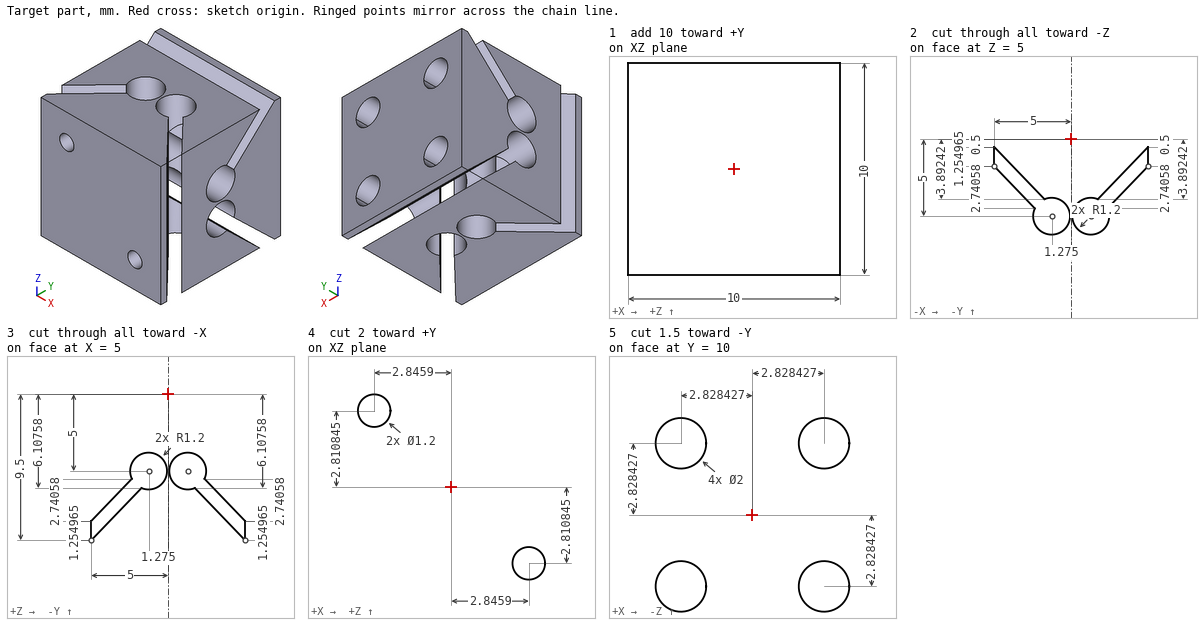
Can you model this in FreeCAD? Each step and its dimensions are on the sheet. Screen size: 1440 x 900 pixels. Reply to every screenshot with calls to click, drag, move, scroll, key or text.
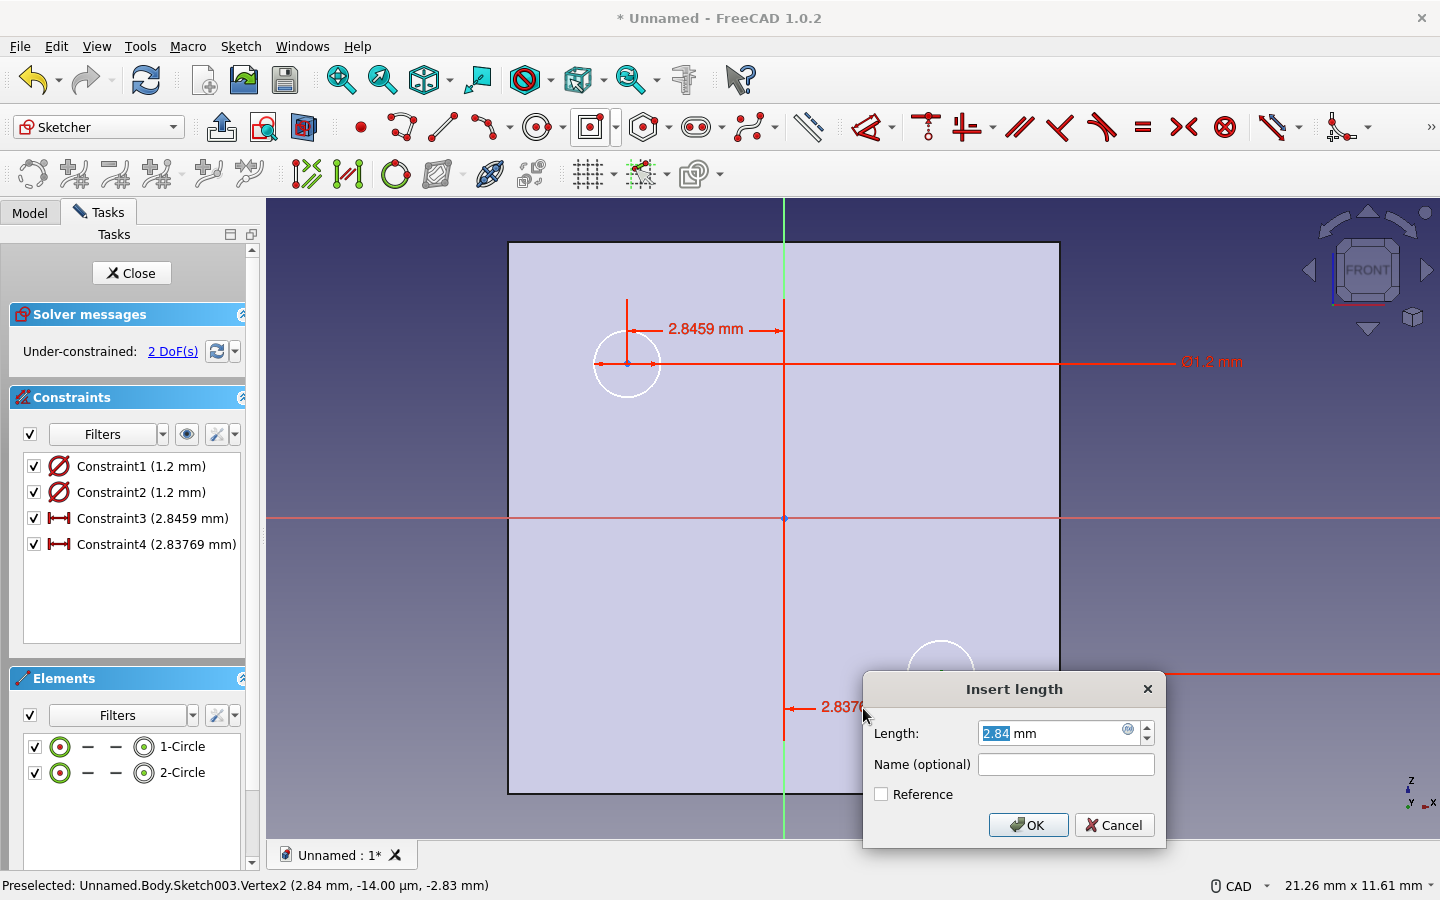
text(2.8459)
key(Return)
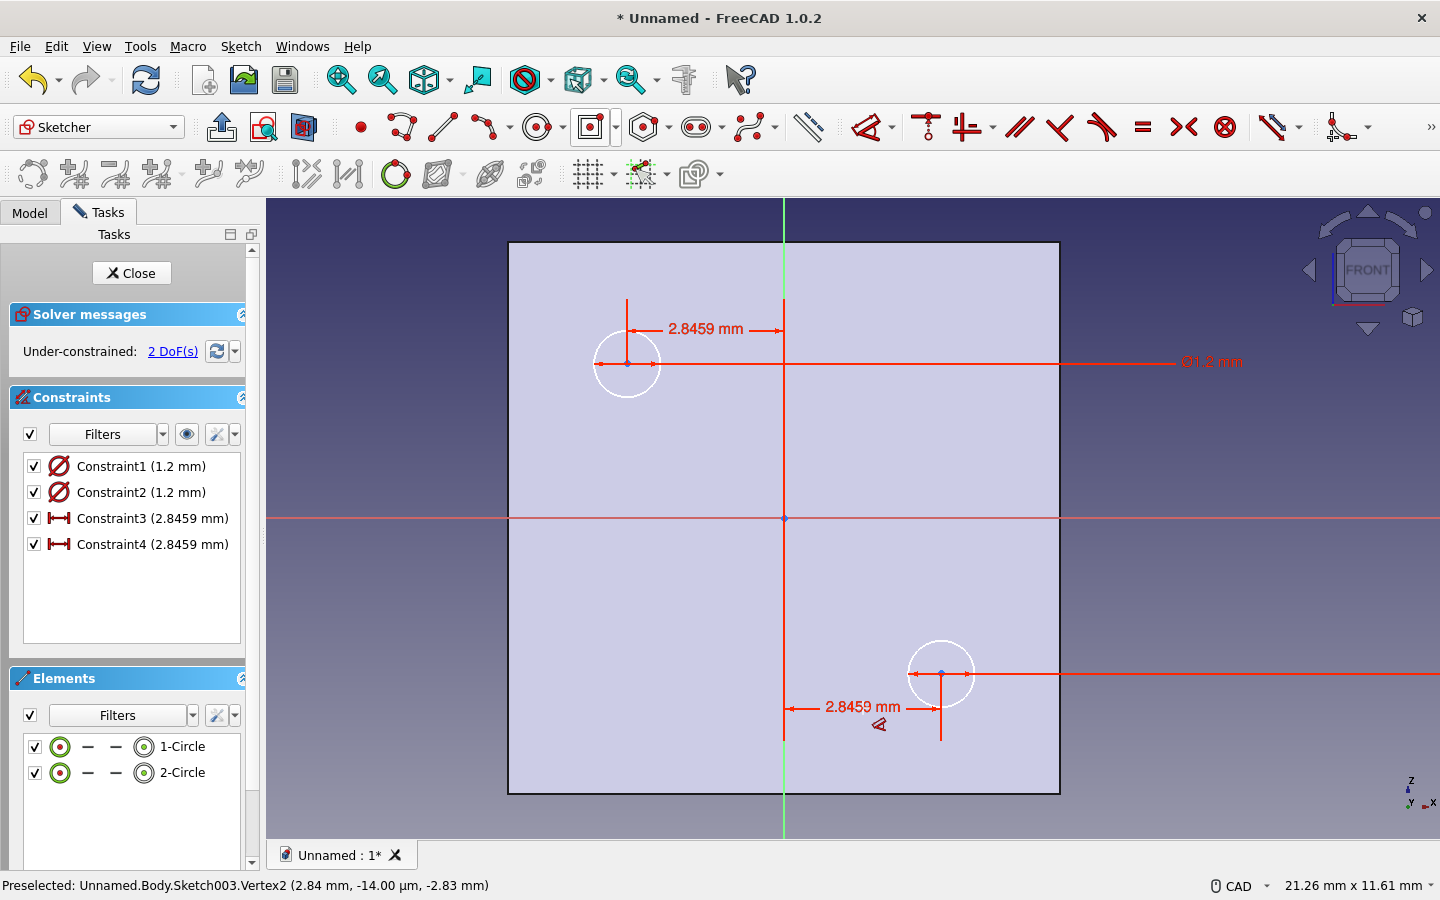
click(627, 364)
click(593, 441)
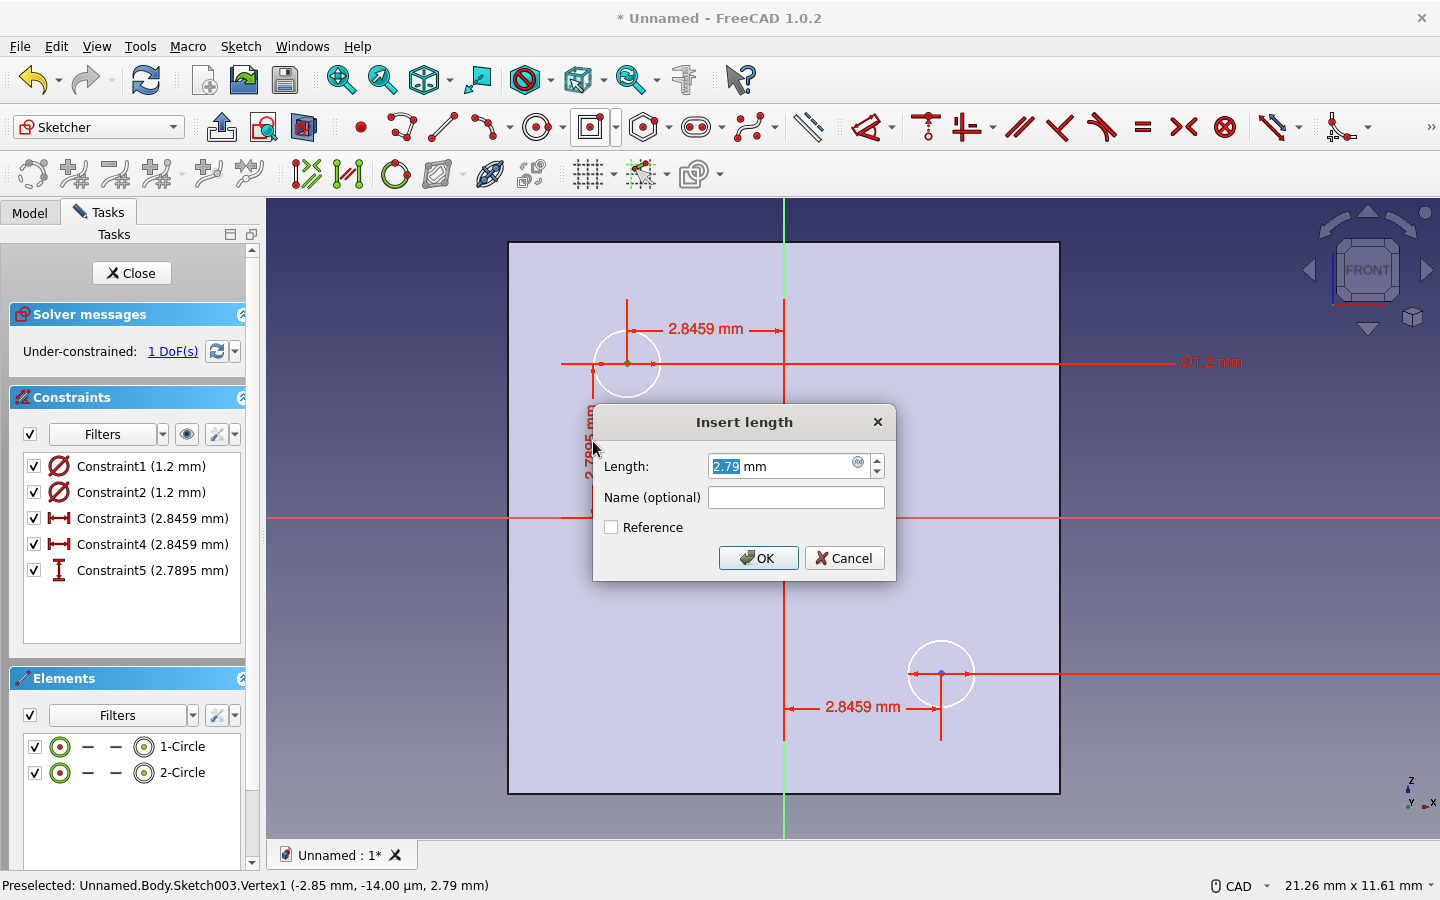
text(2.810845)
key(Return)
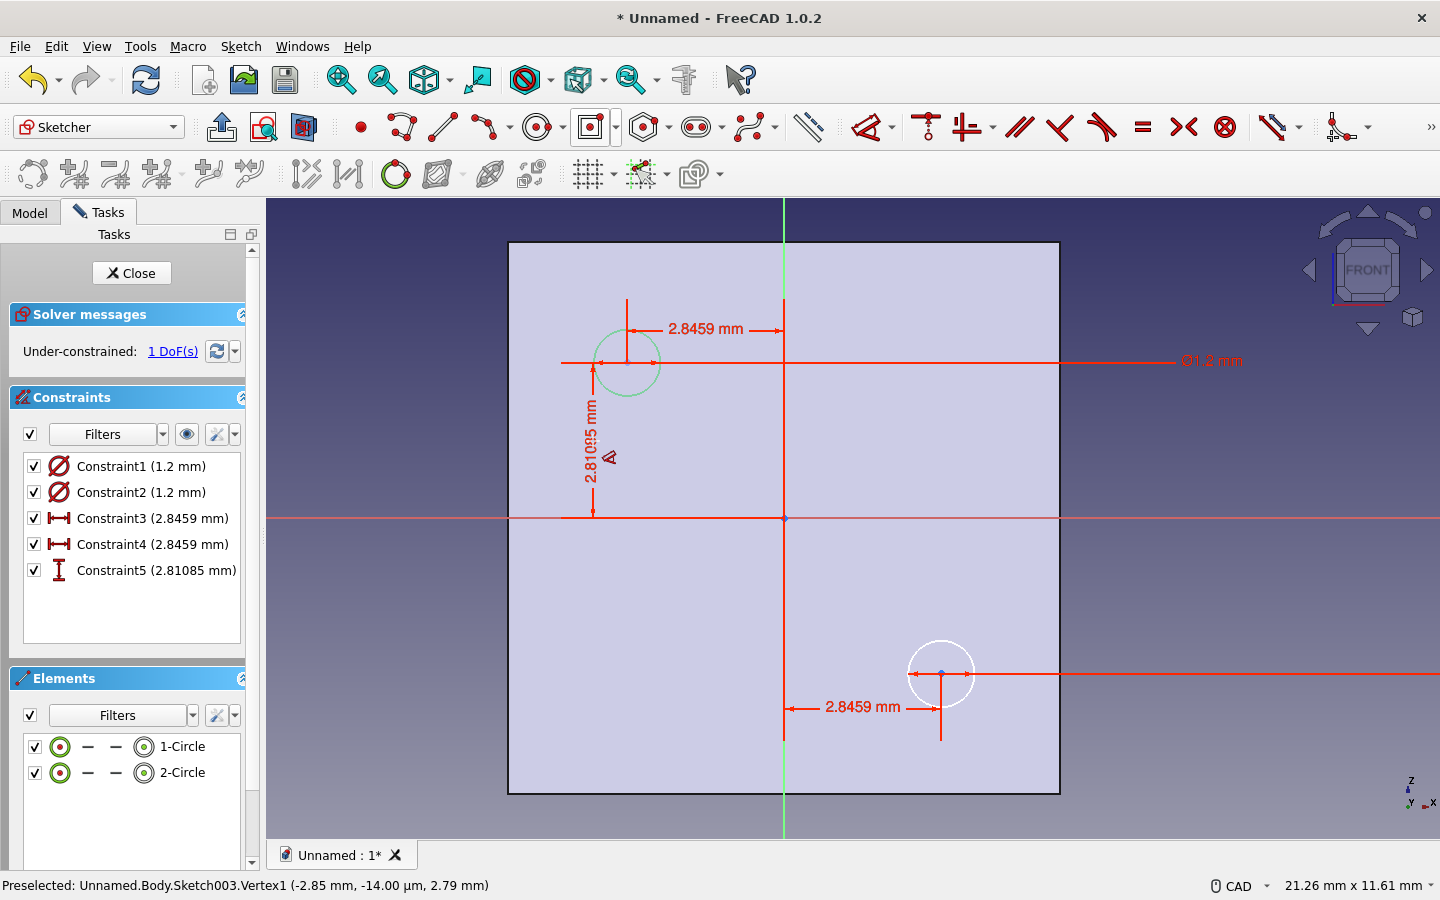
click(941, 674)
click(975, 596)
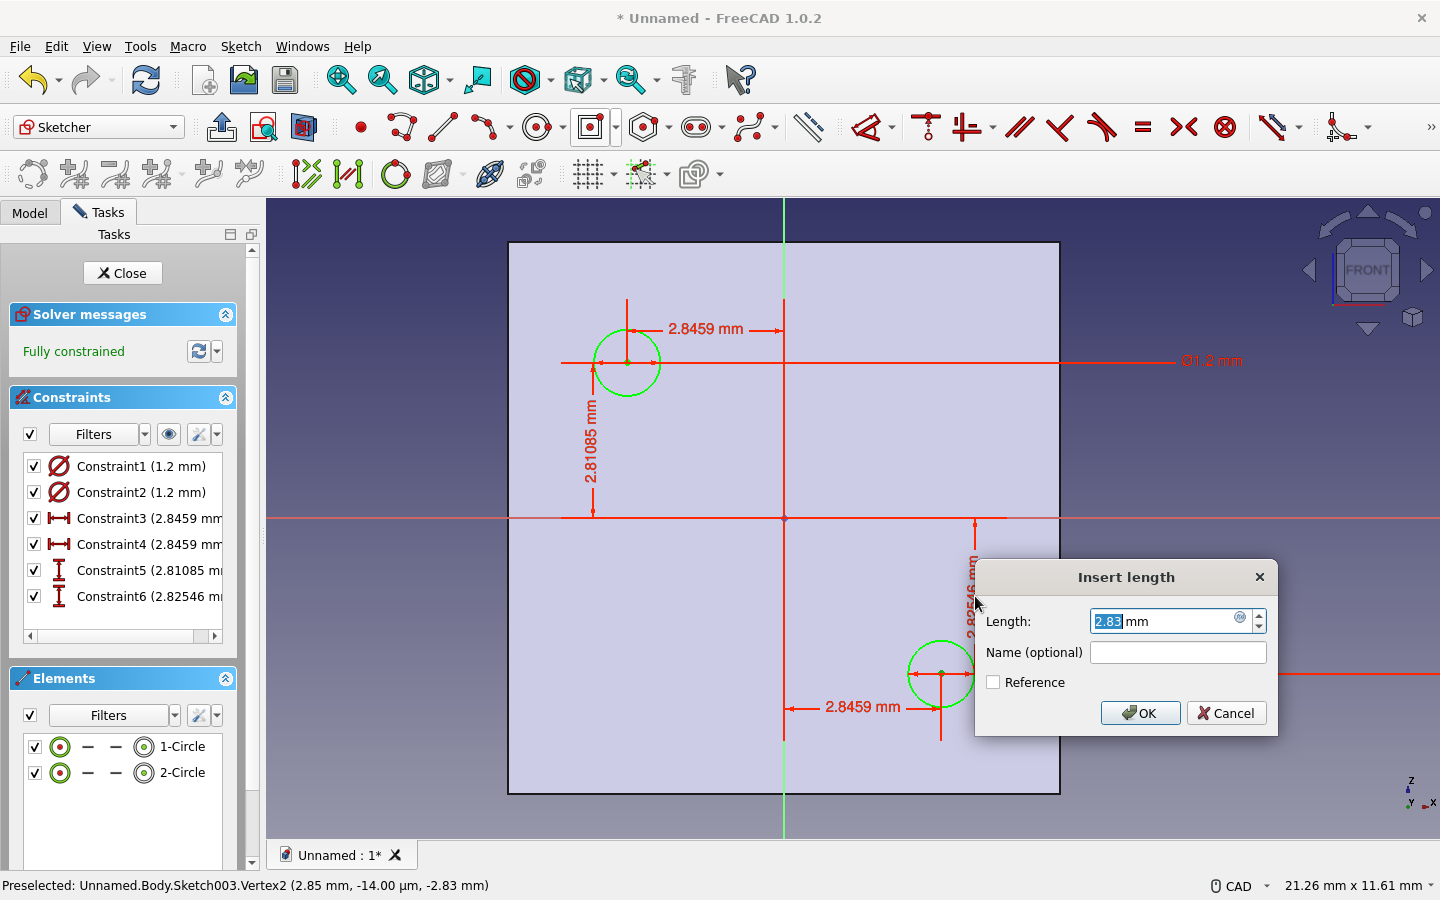
text(2.810845)
key(Return)
key(Escape)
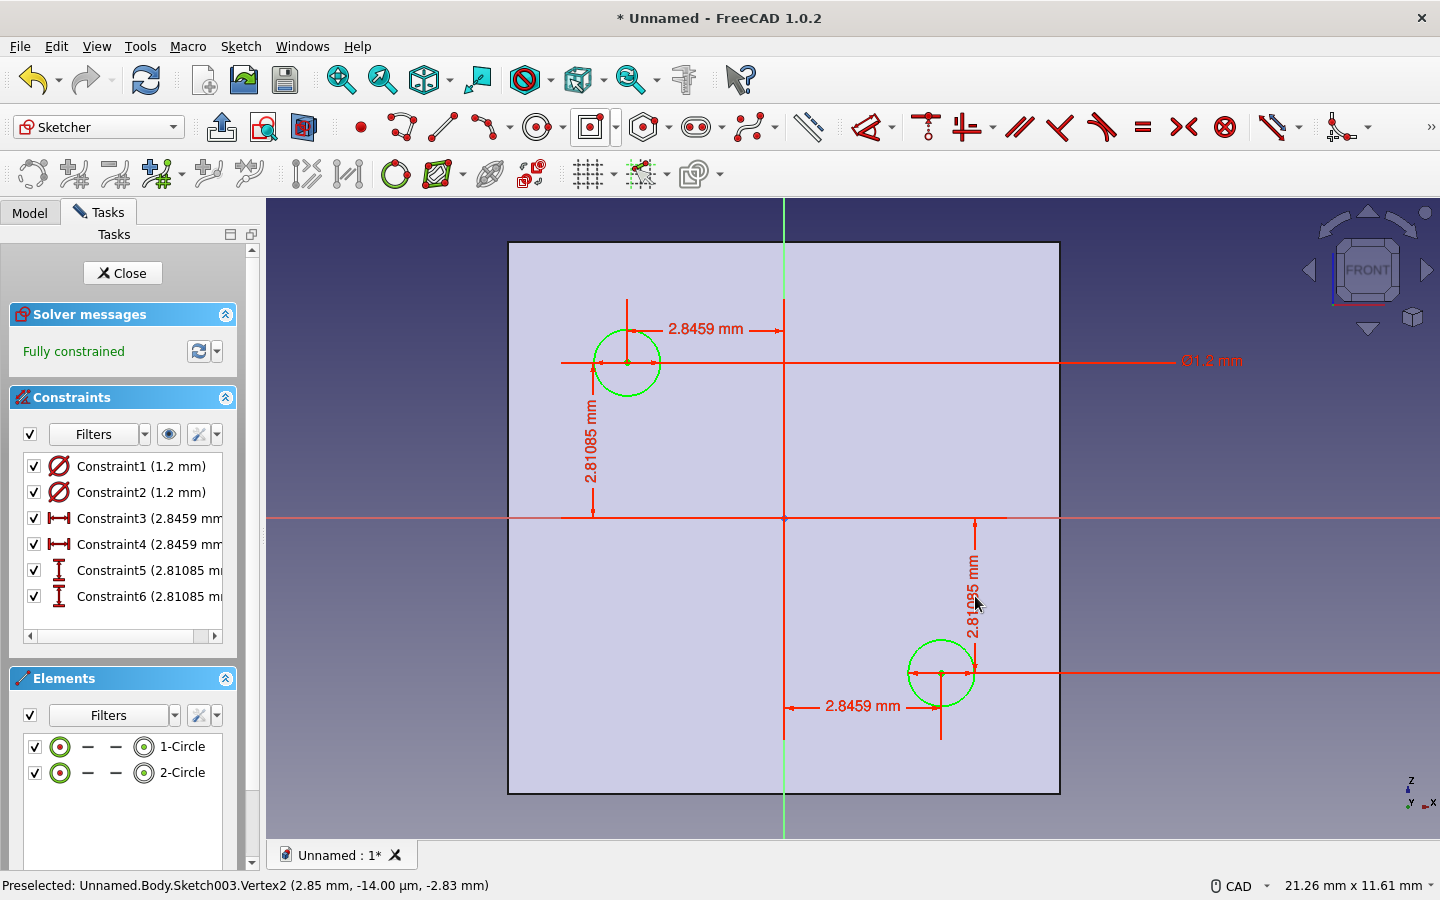
click(123, 273)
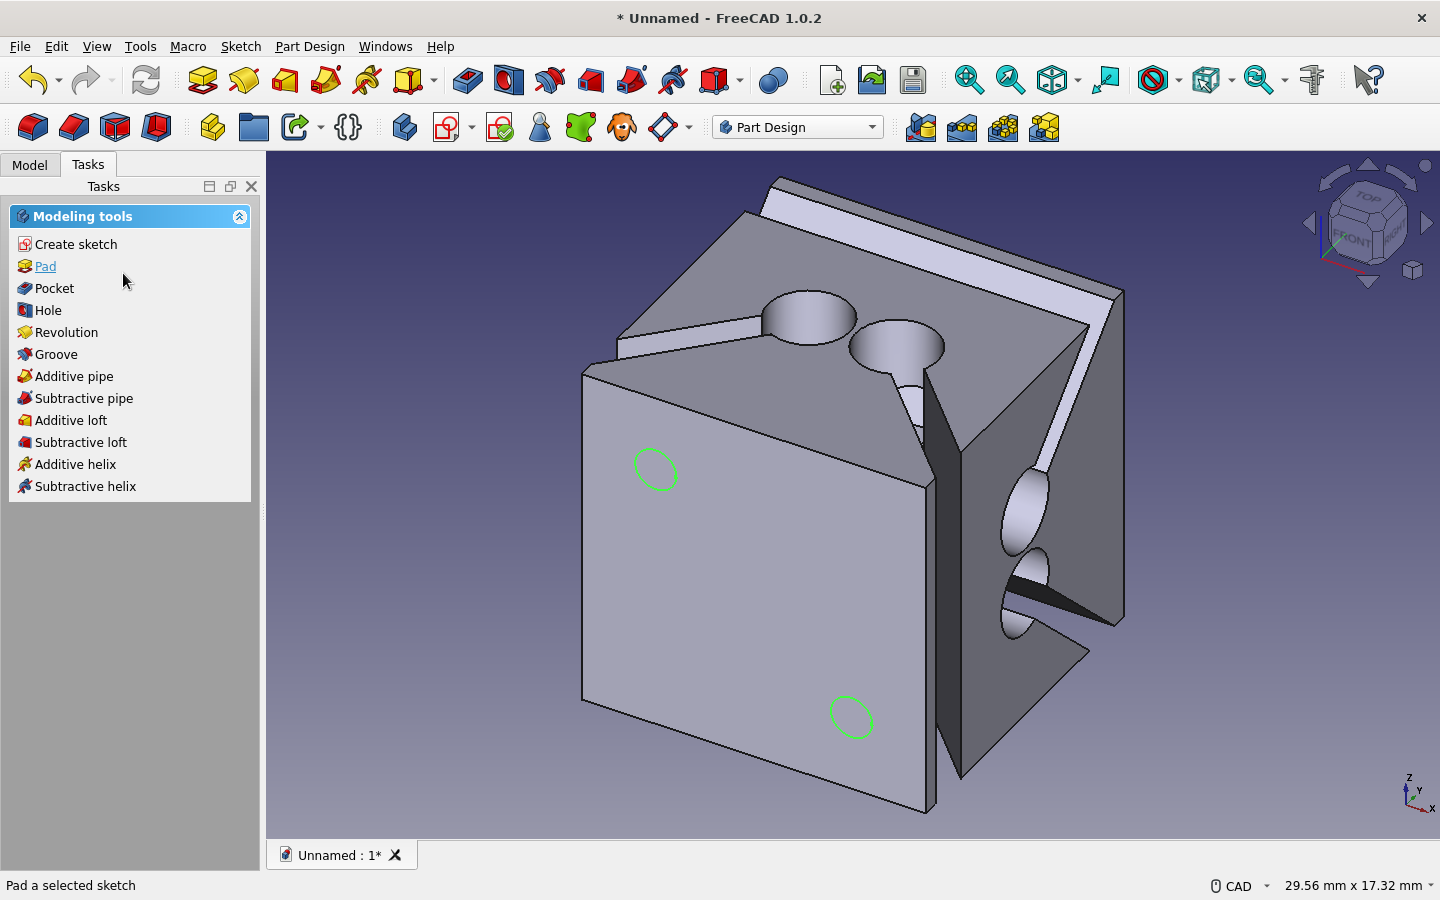
click(468, 80)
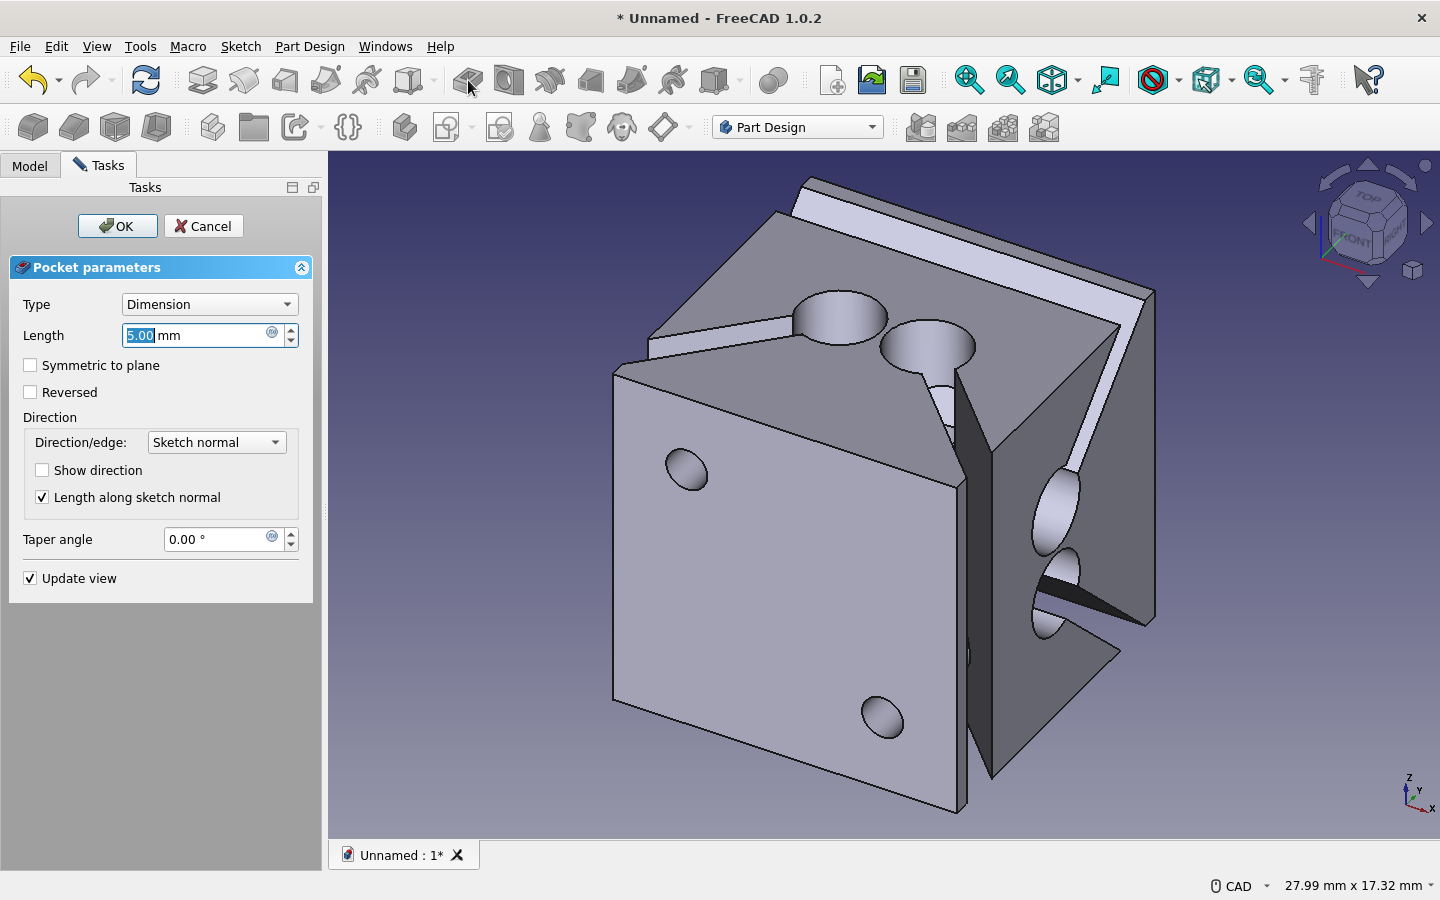
text(2)
key(Tab)